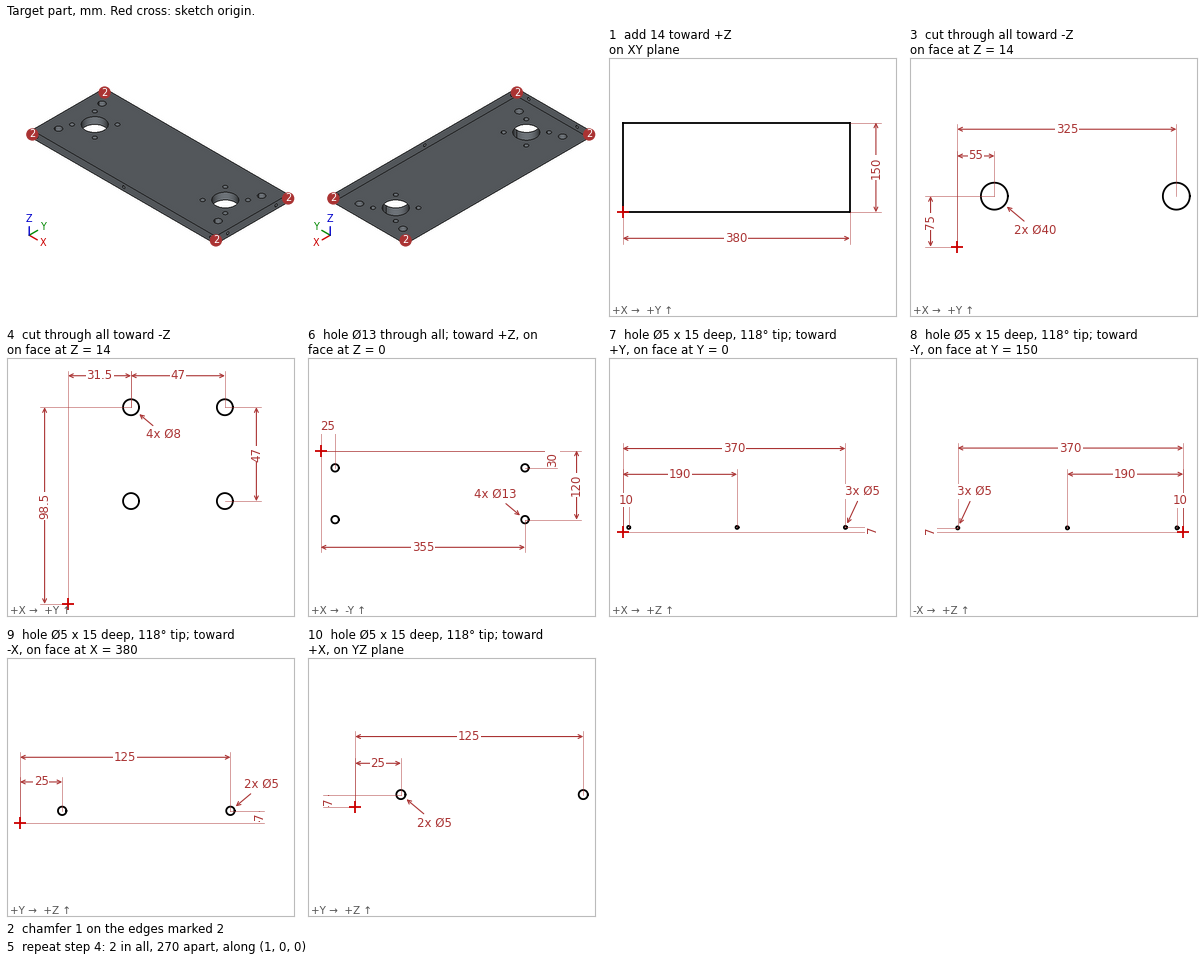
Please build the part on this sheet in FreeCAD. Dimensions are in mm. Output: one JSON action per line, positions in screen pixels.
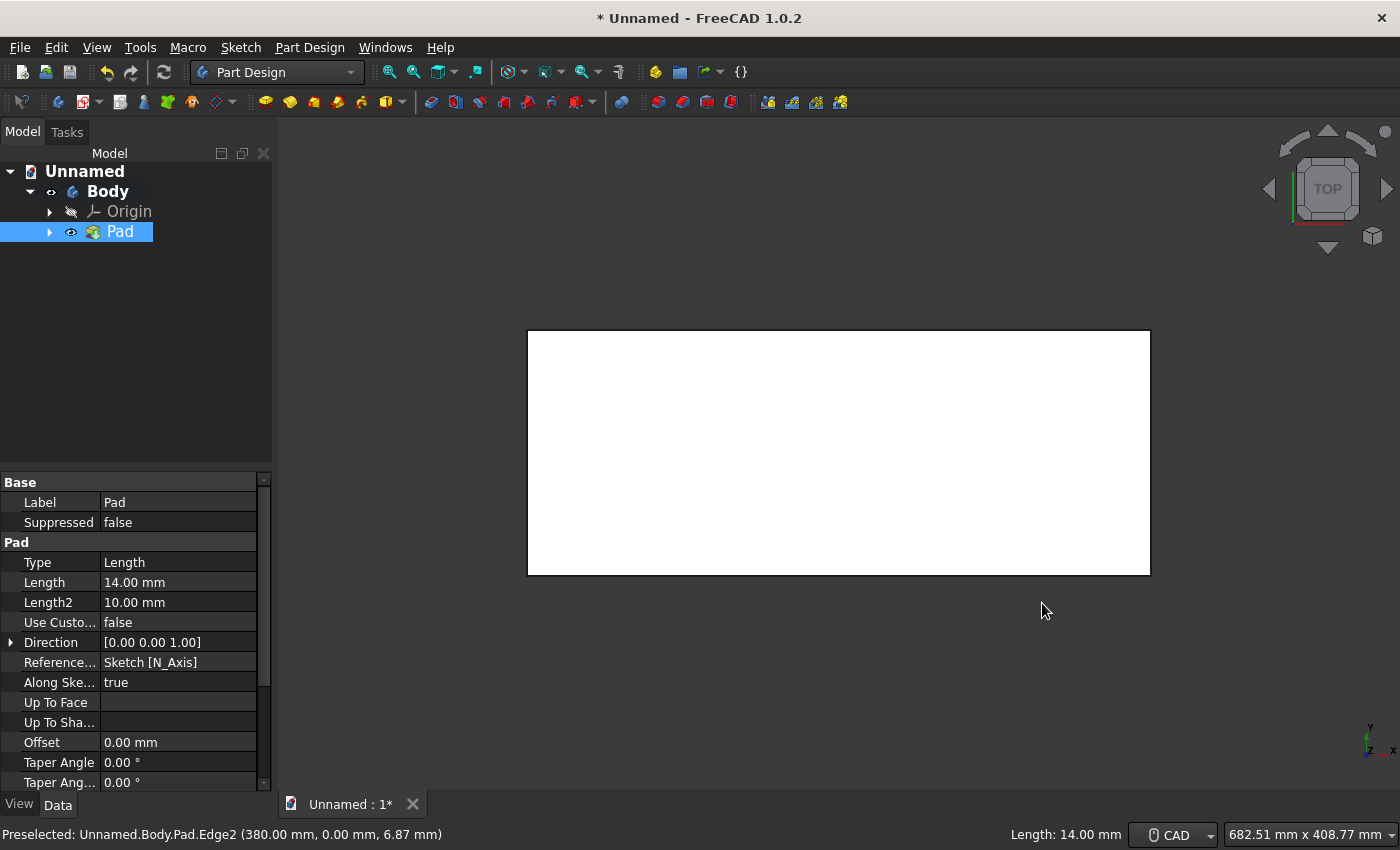
{"action": "key", "text": "1"}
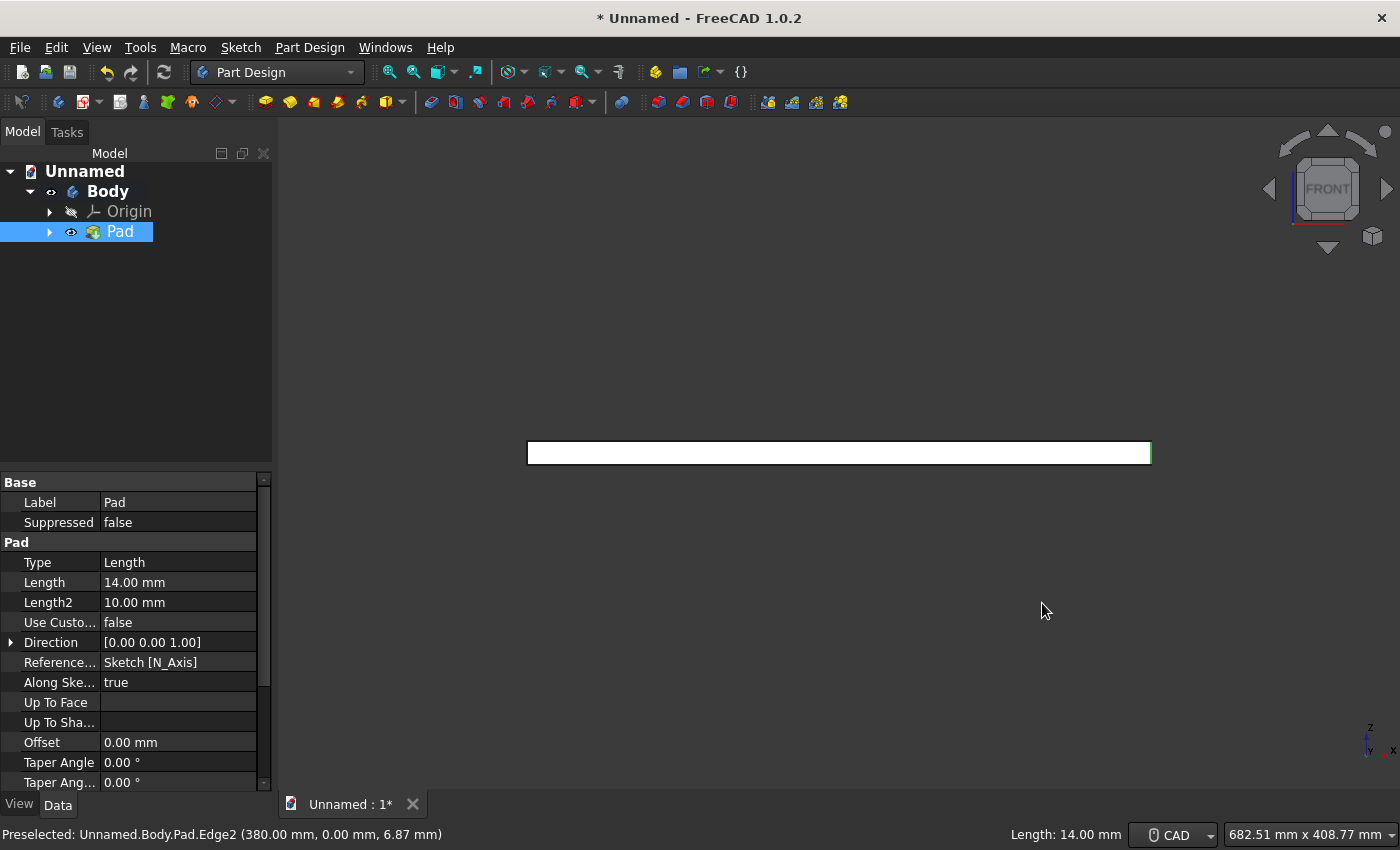
{"action": "left_click", "coordinate": [527, 452], "text": "ctrl"}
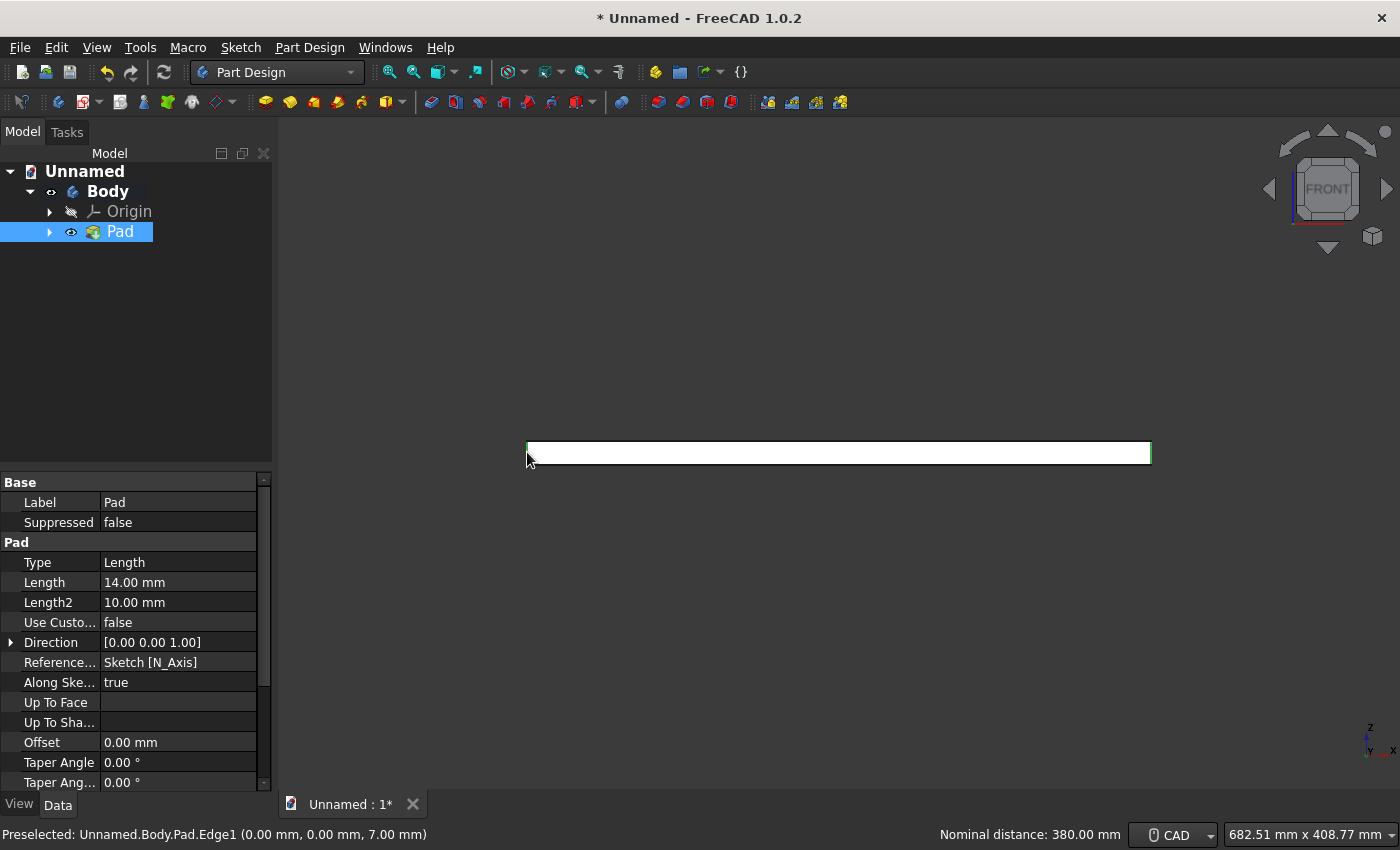
{"action": "key", "text": "3"}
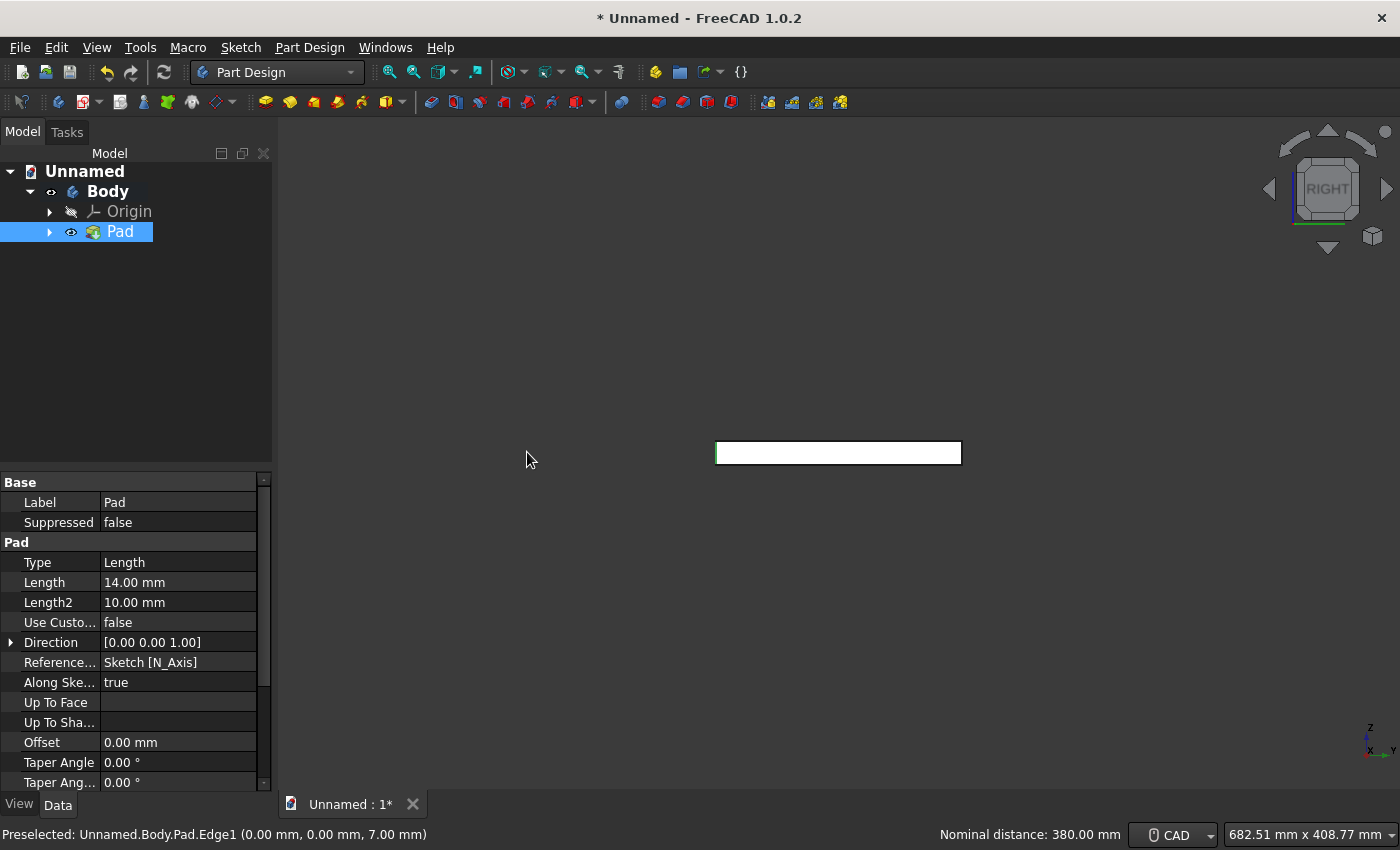
{"action": "key", "text": "v f"}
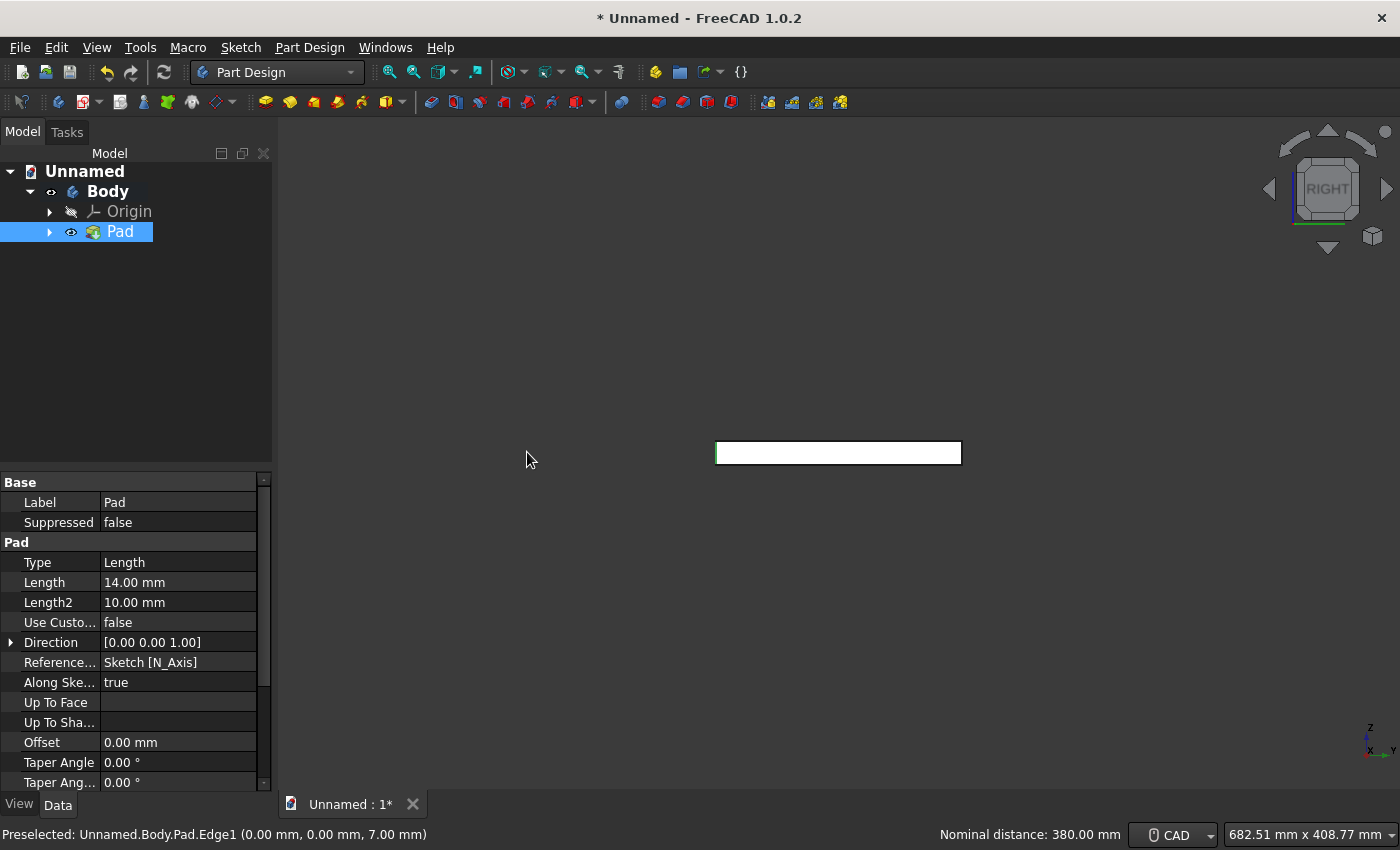
{"action": "left_click", "coordinate": [962, 452], "text": "ctrl"}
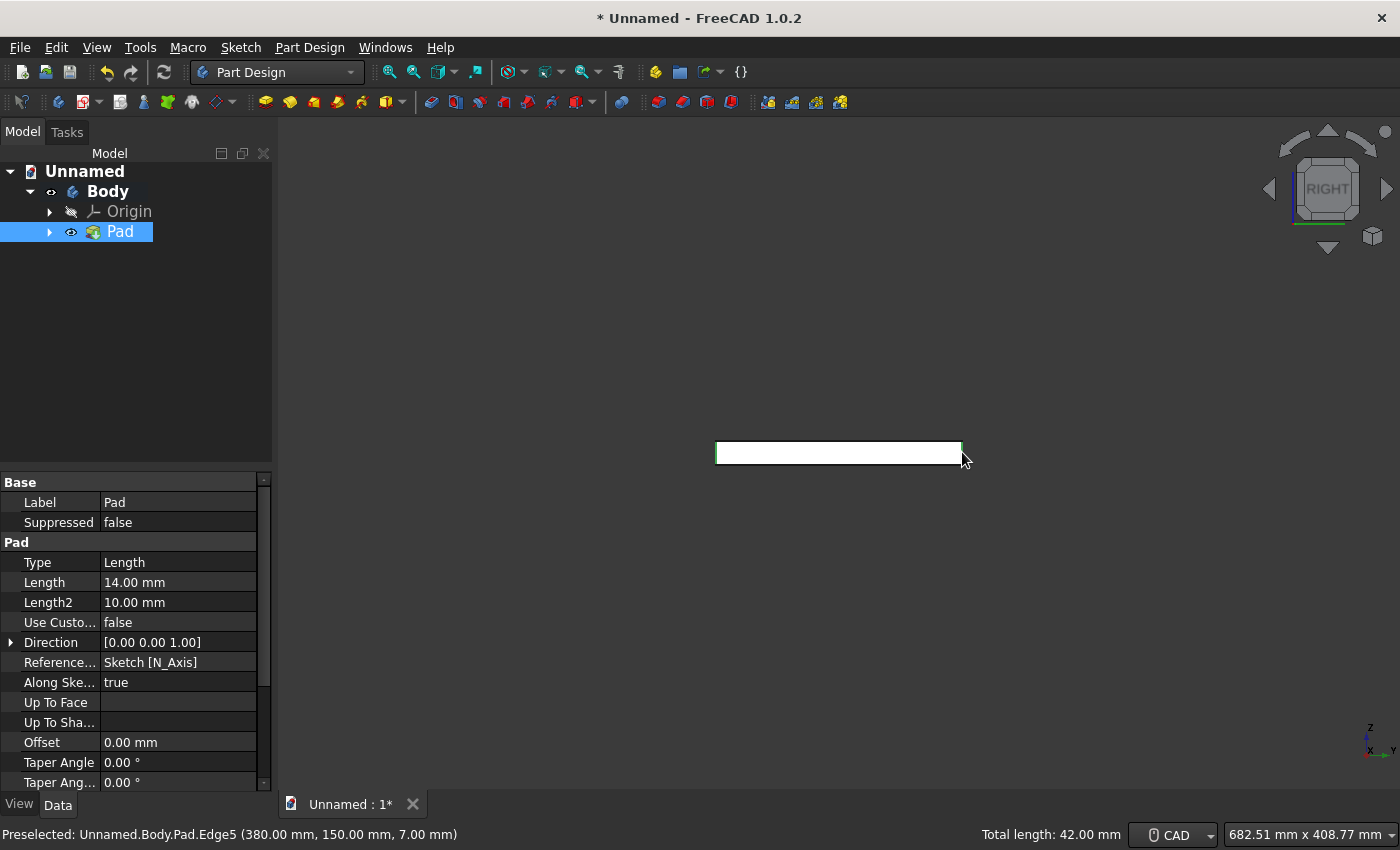
{"action": "key", "text": "5"}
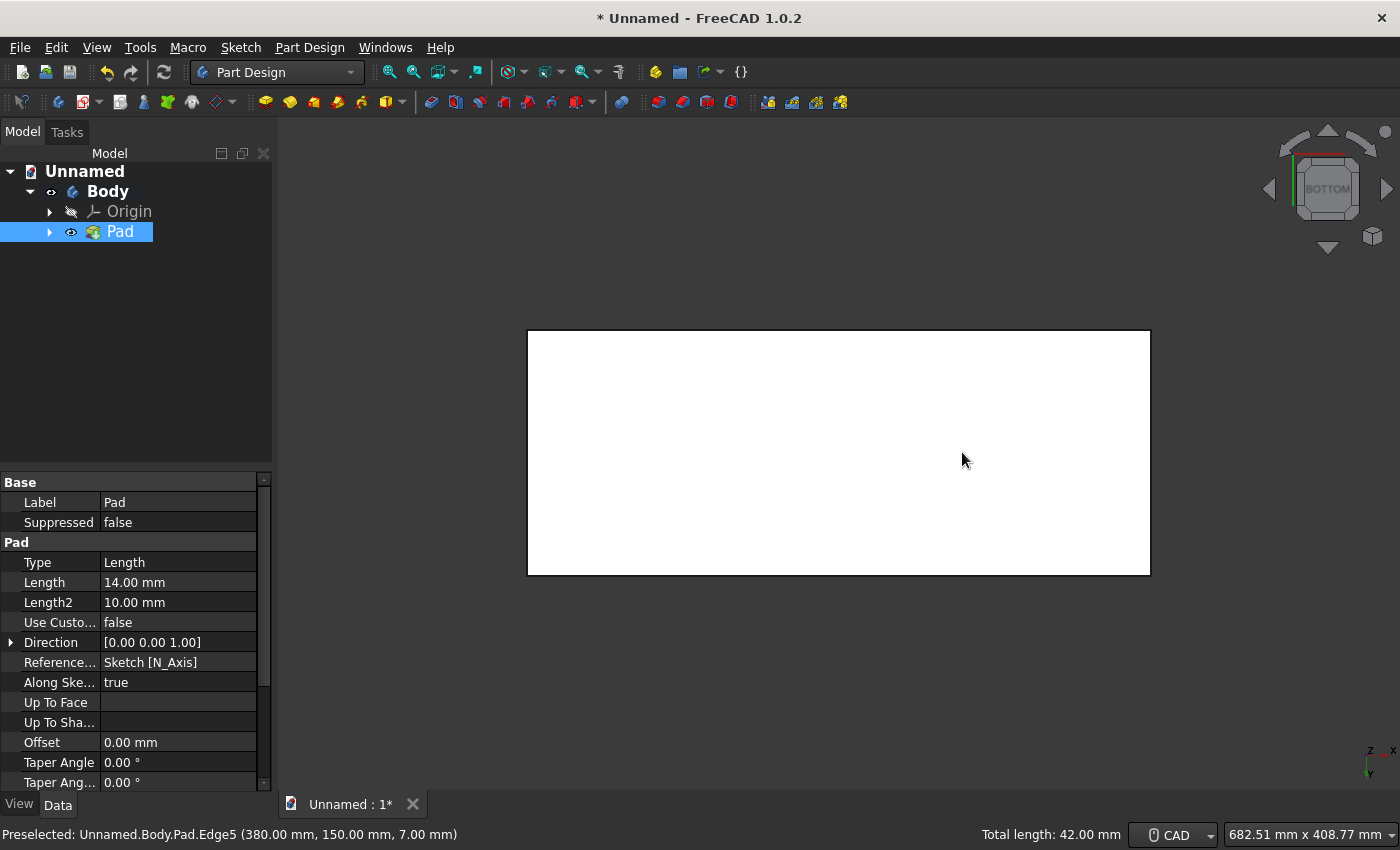
{"action": "key", "text": "4"}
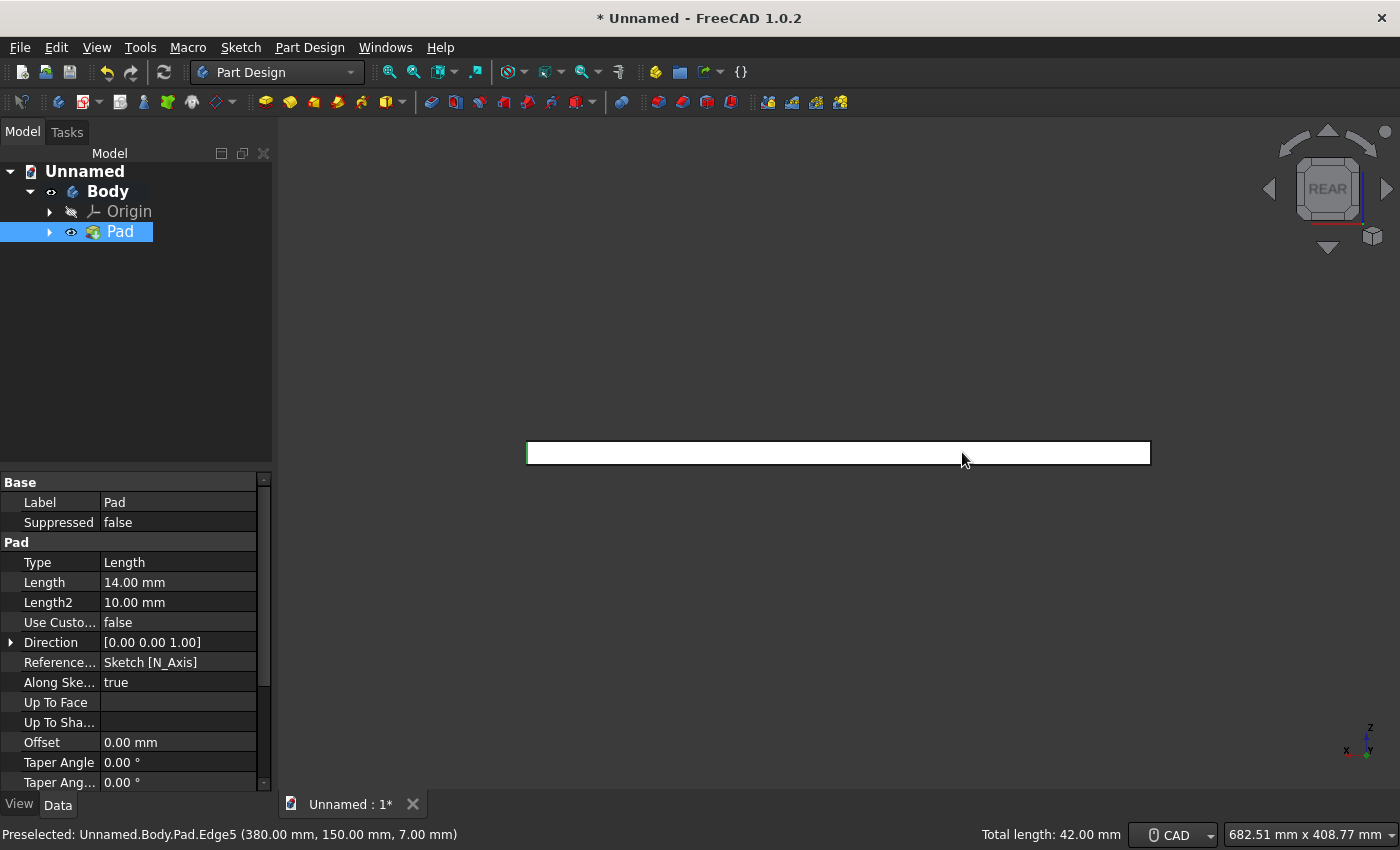
{"action": "left_click", "coordinate": [1151, 452], "text": "ctrl"}